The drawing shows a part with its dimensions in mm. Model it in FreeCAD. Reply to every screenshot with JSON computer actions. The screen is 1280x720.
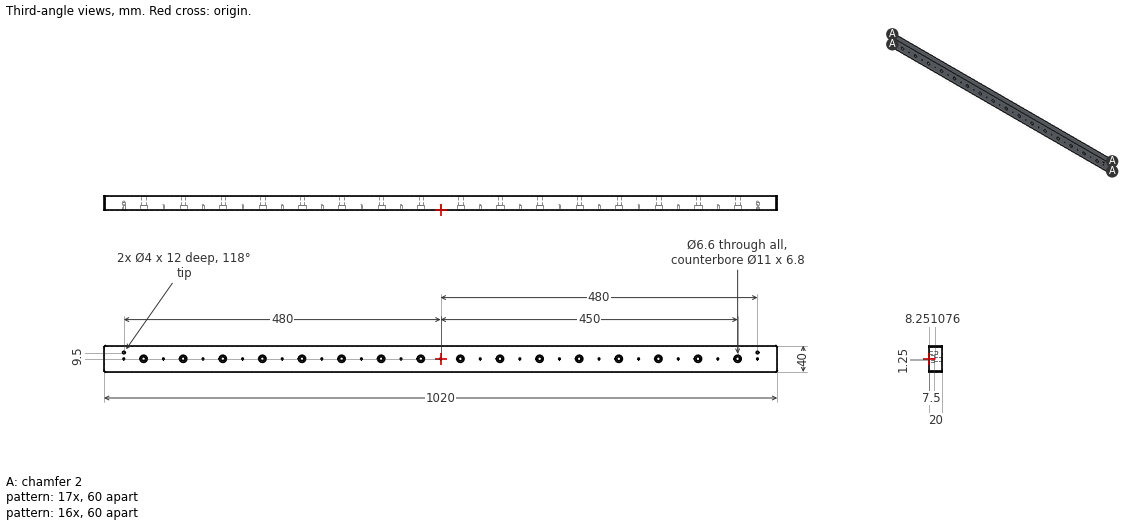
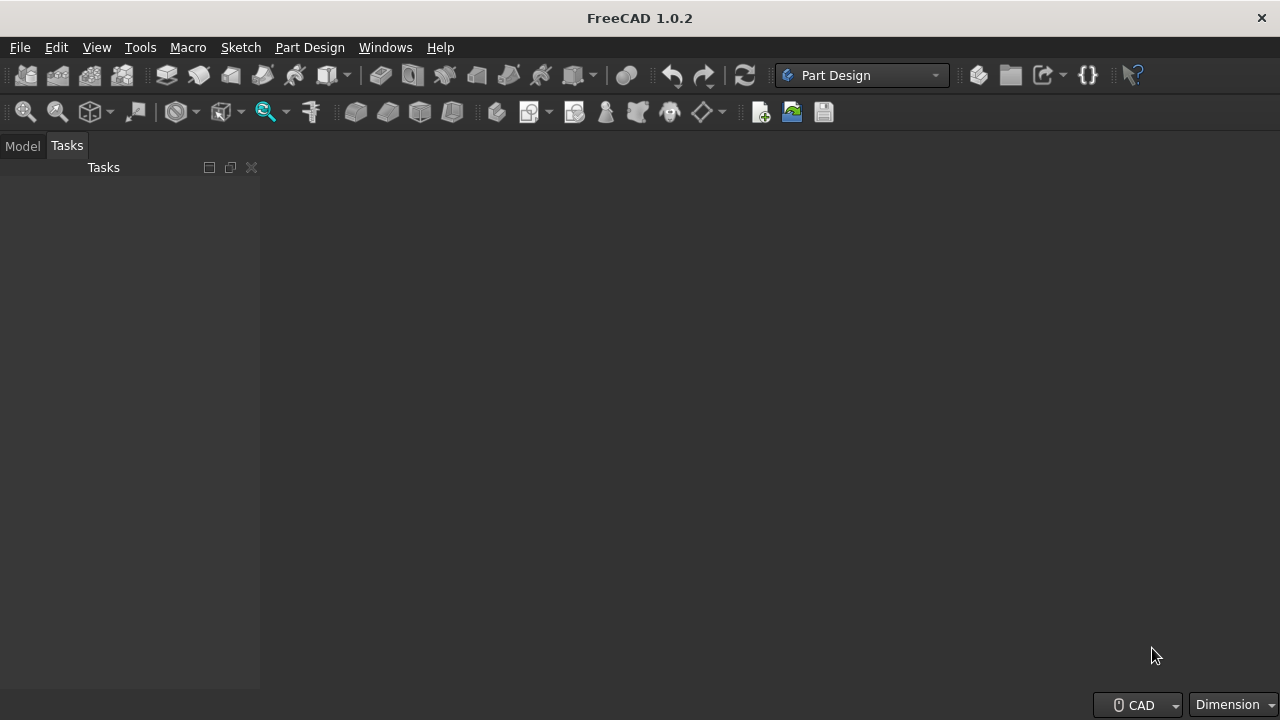
{"action": "left_click", "coordinate": [760, 112]}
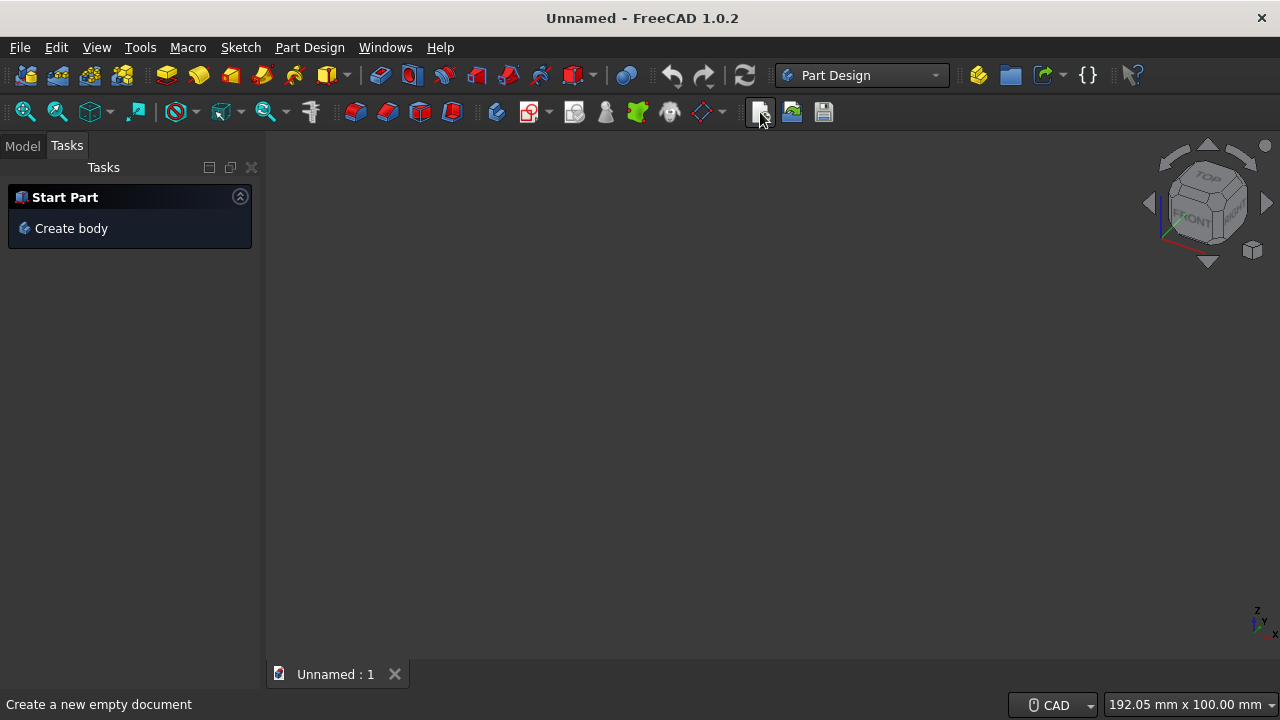
{"action": "left_click", "coordinate": [530, 112]}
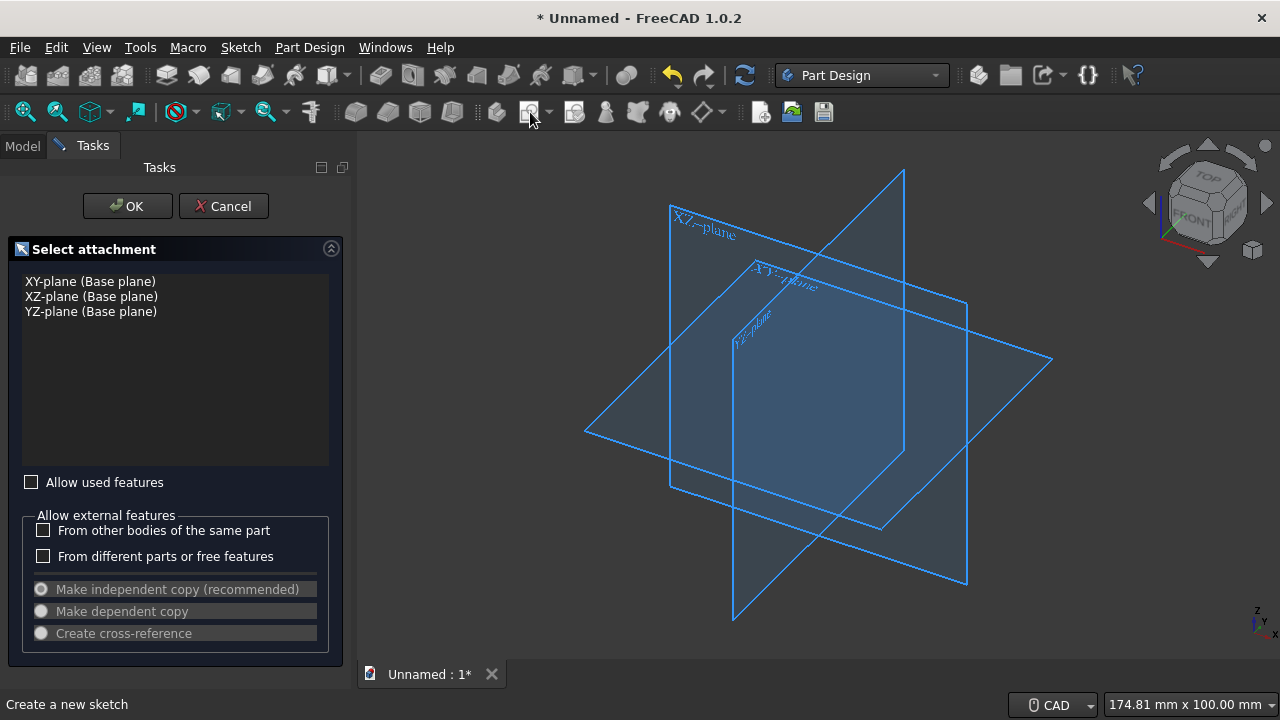
{"action": "left_click", "coordinate": [82, 296]}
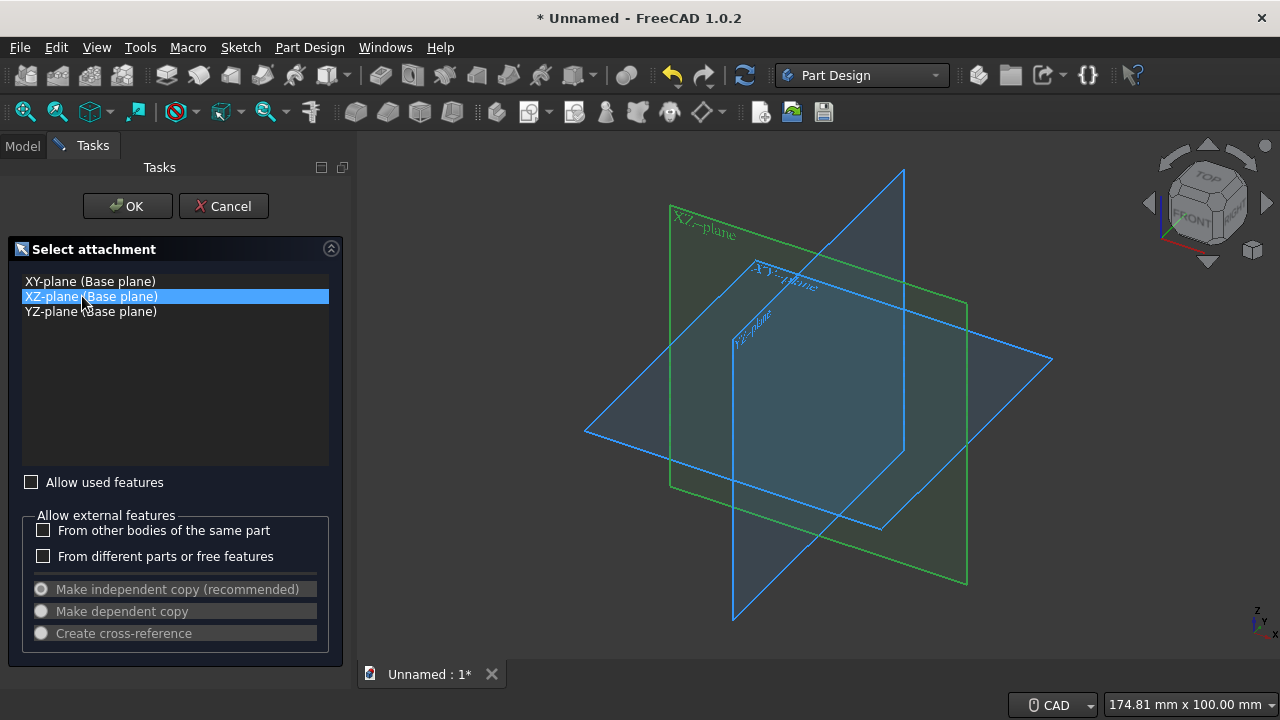
{"action": "left_click", "coordinate": [128, 206]}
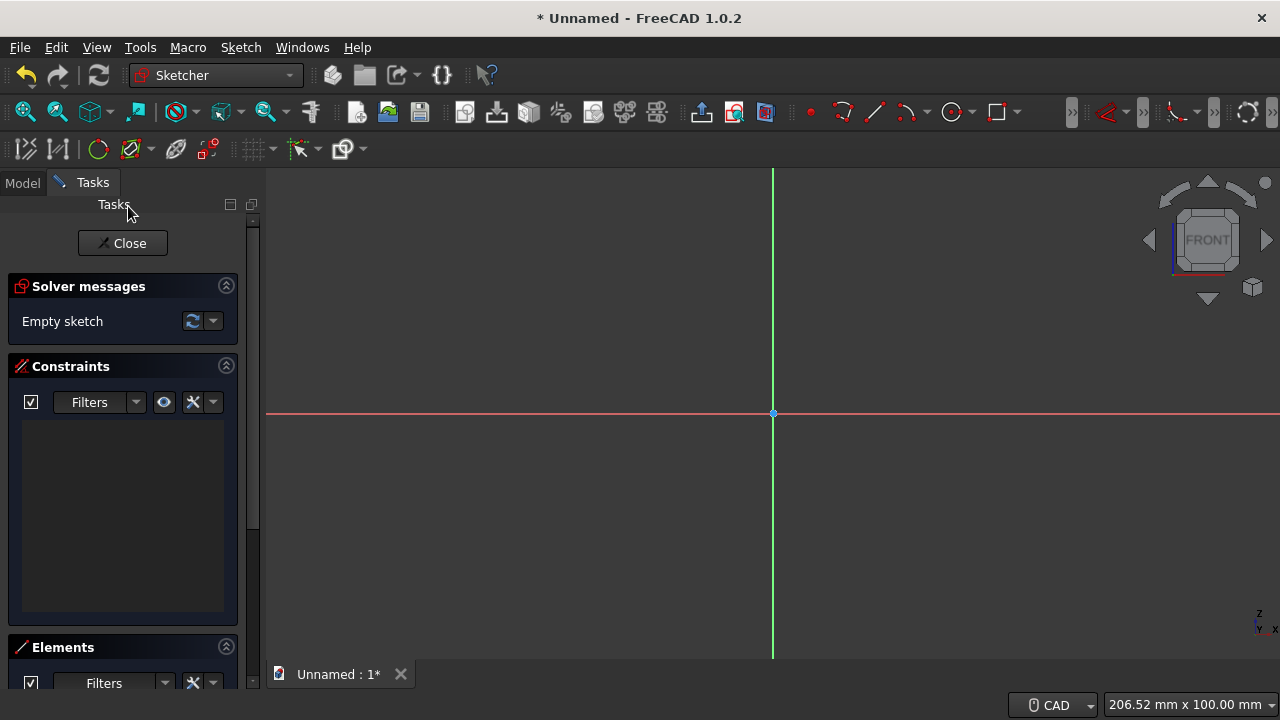
{"action": "scroll", "coordinate": [696, 414], "scroll_direction": "down", "scroll_amount": 11}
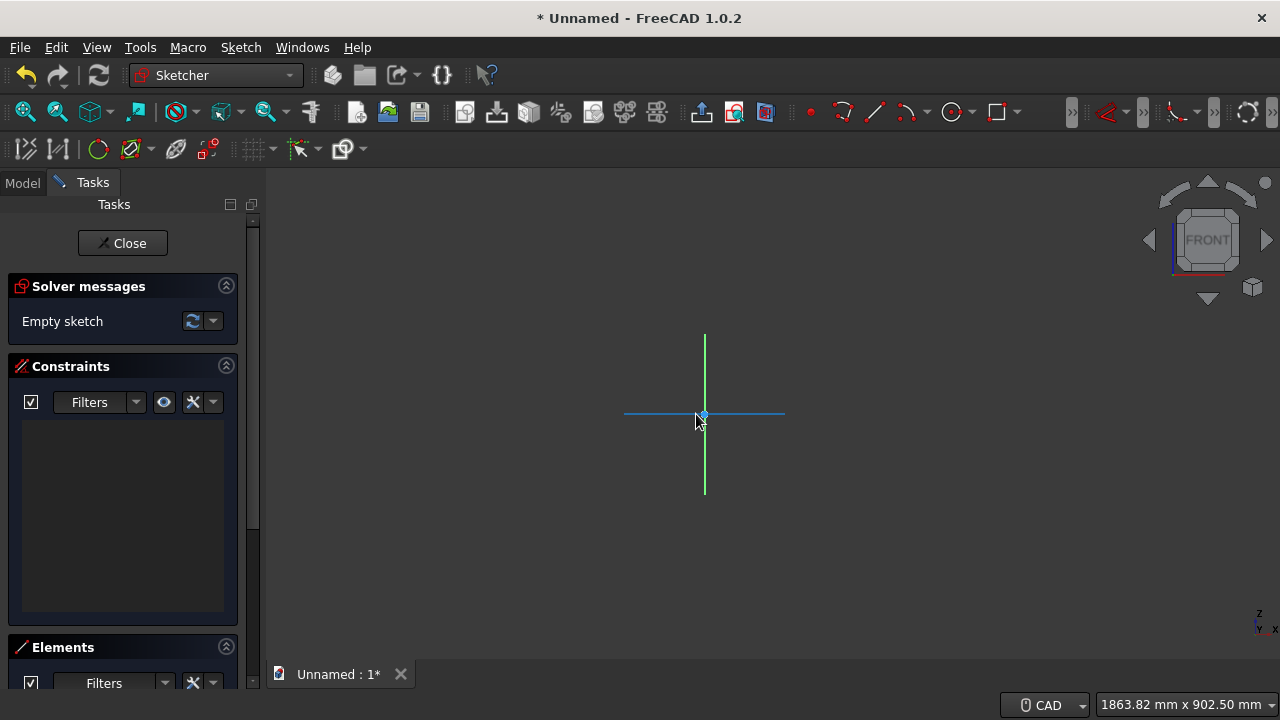
{"action": "key", "text": "g v"}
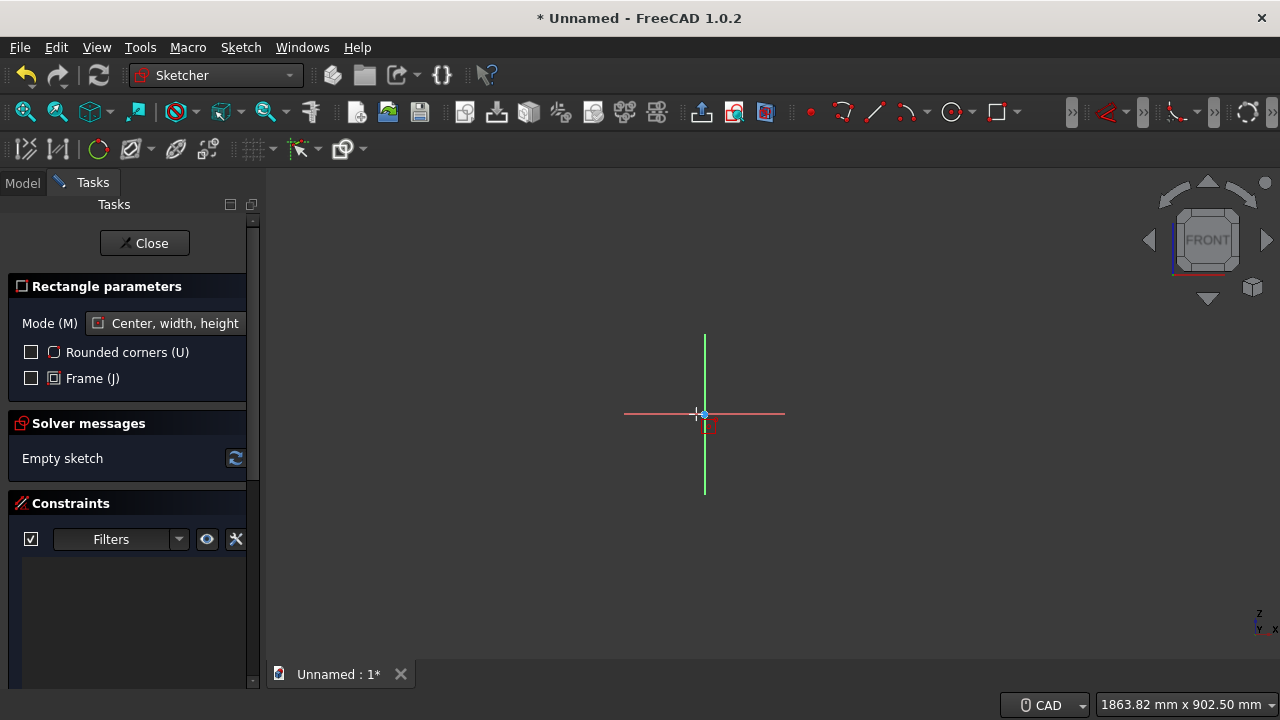
{"action": "scroll", "coordinate": [705, 414], "scroll_direction": "up", "scroll_amount": 2}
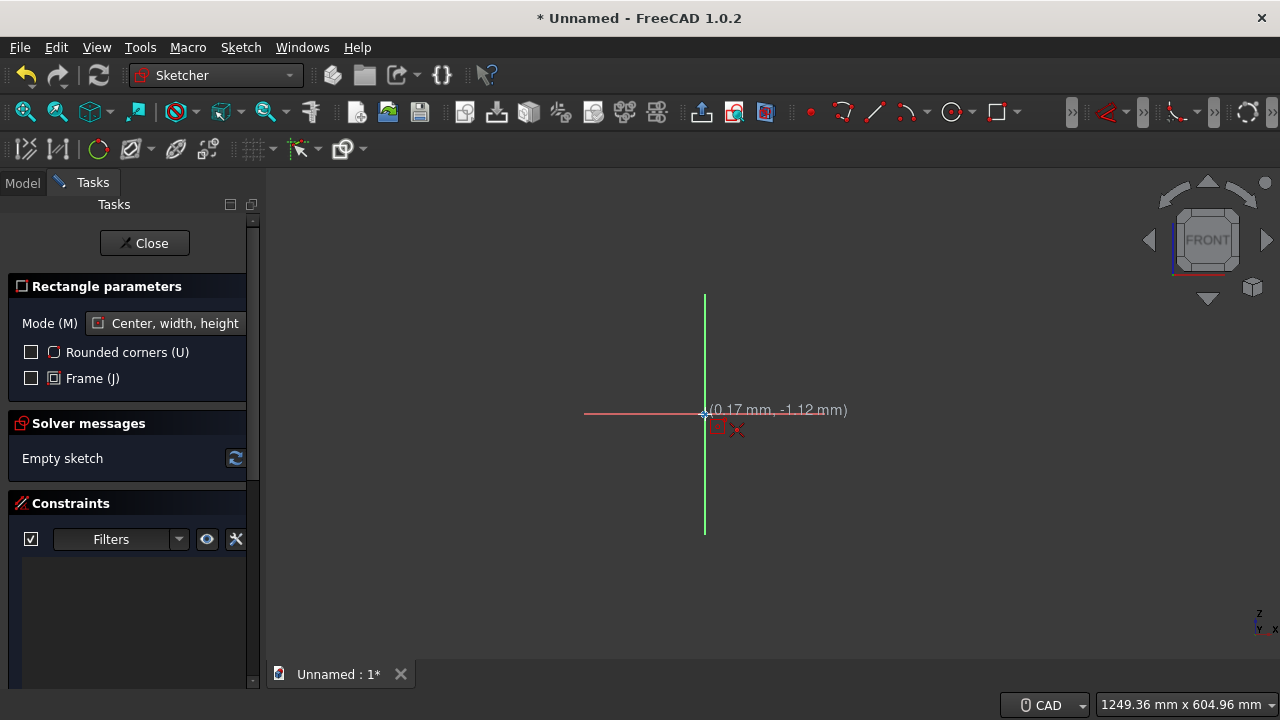
{"action": "left_click", "coordinate": [705, 414]}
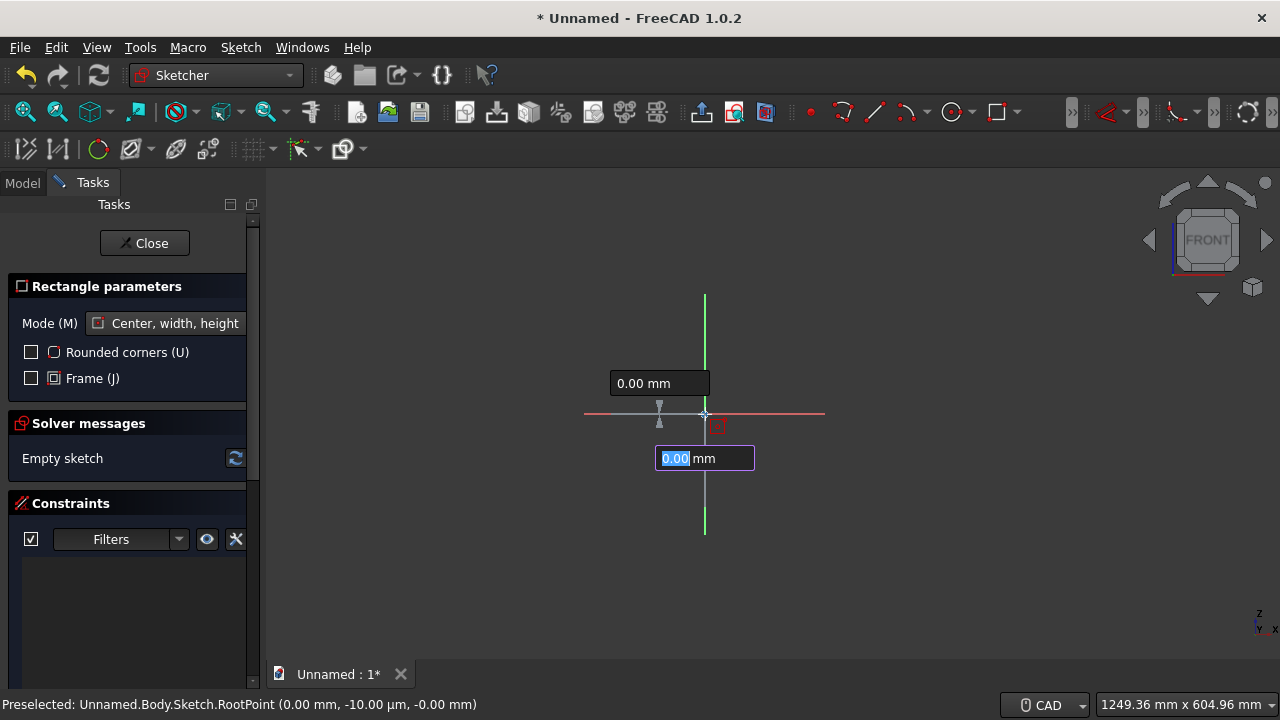
{"action": "scroll", "coordinate": [704, 412], "scroll_direction": "down", "scroll_amount": 2}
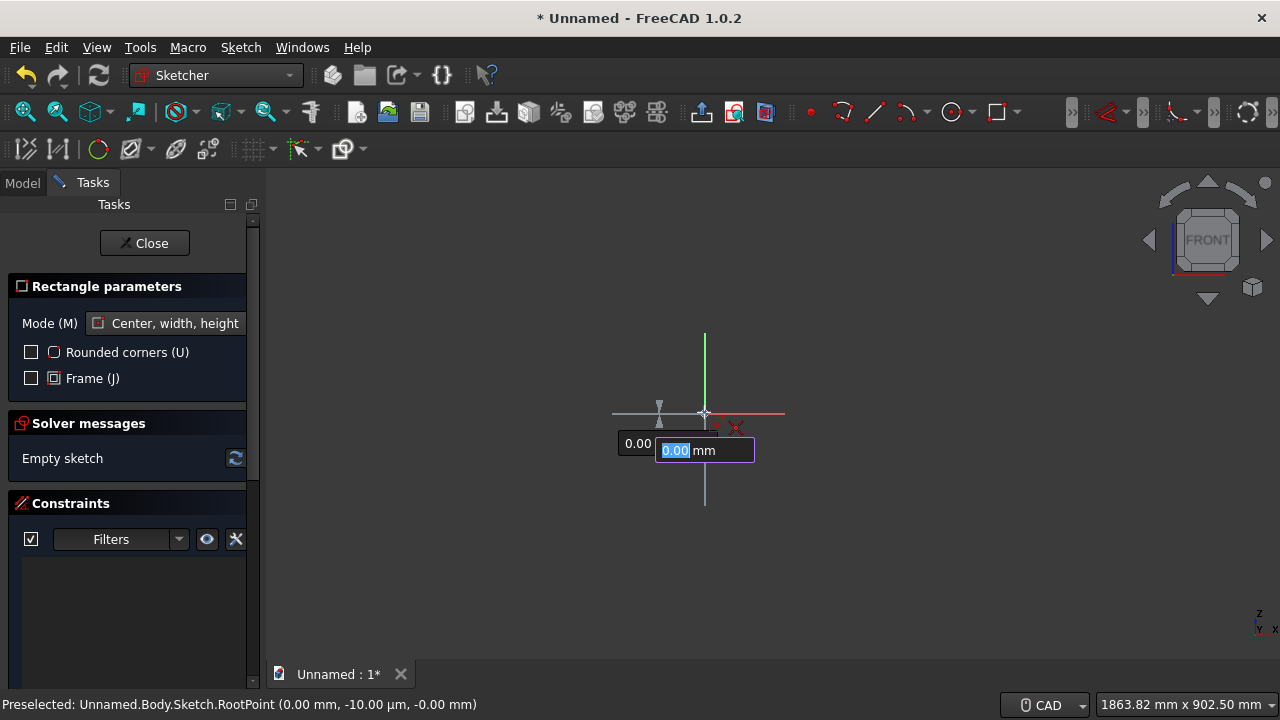
{"action": "scroll", "coordinate": [982, 403], "scroll_direction": "up", "scroll_amount": 2}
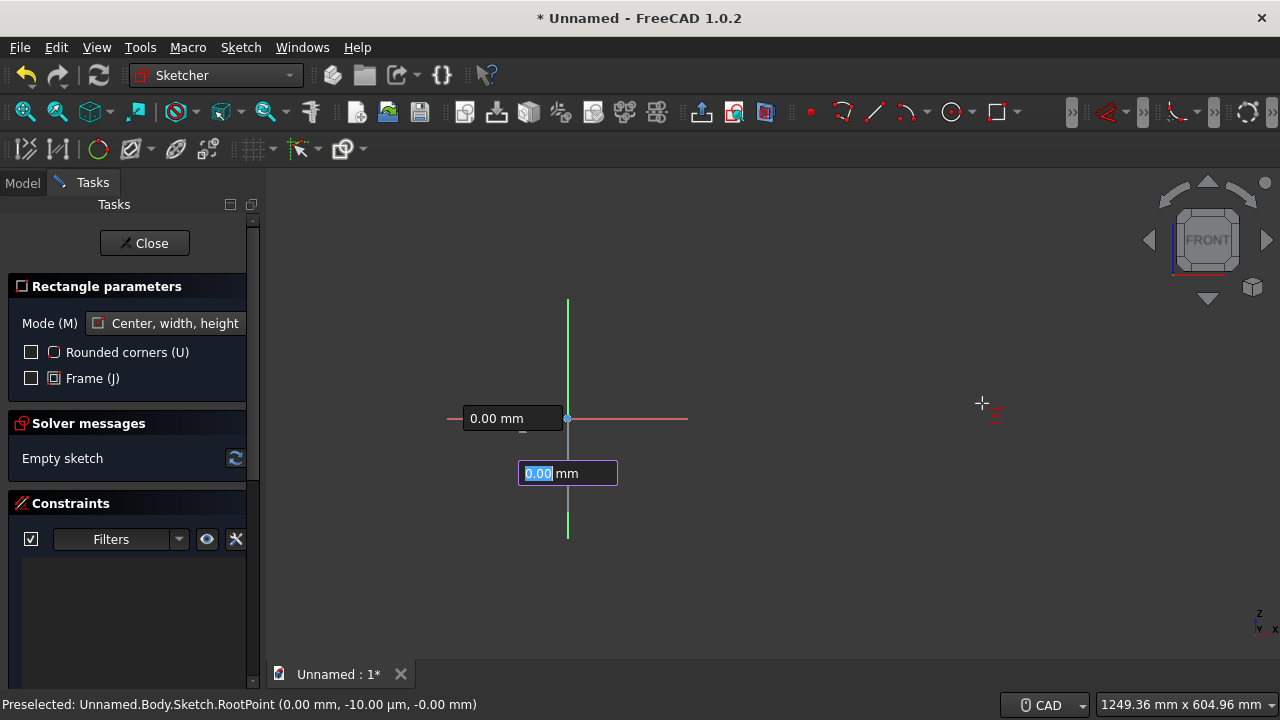
{"action": "left_click", "coordinate": [982, 403]}
{"action": "key", "text": "Escape"}